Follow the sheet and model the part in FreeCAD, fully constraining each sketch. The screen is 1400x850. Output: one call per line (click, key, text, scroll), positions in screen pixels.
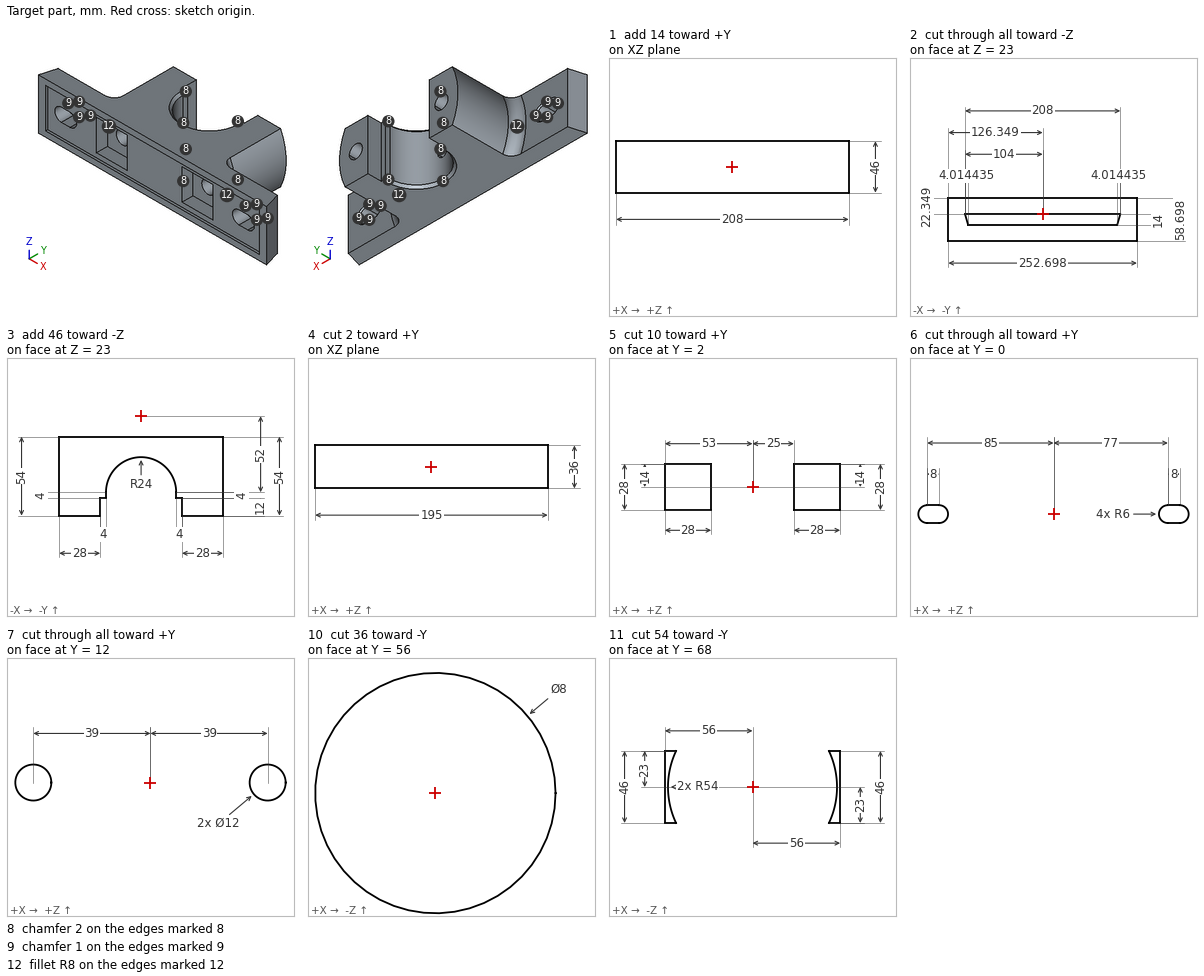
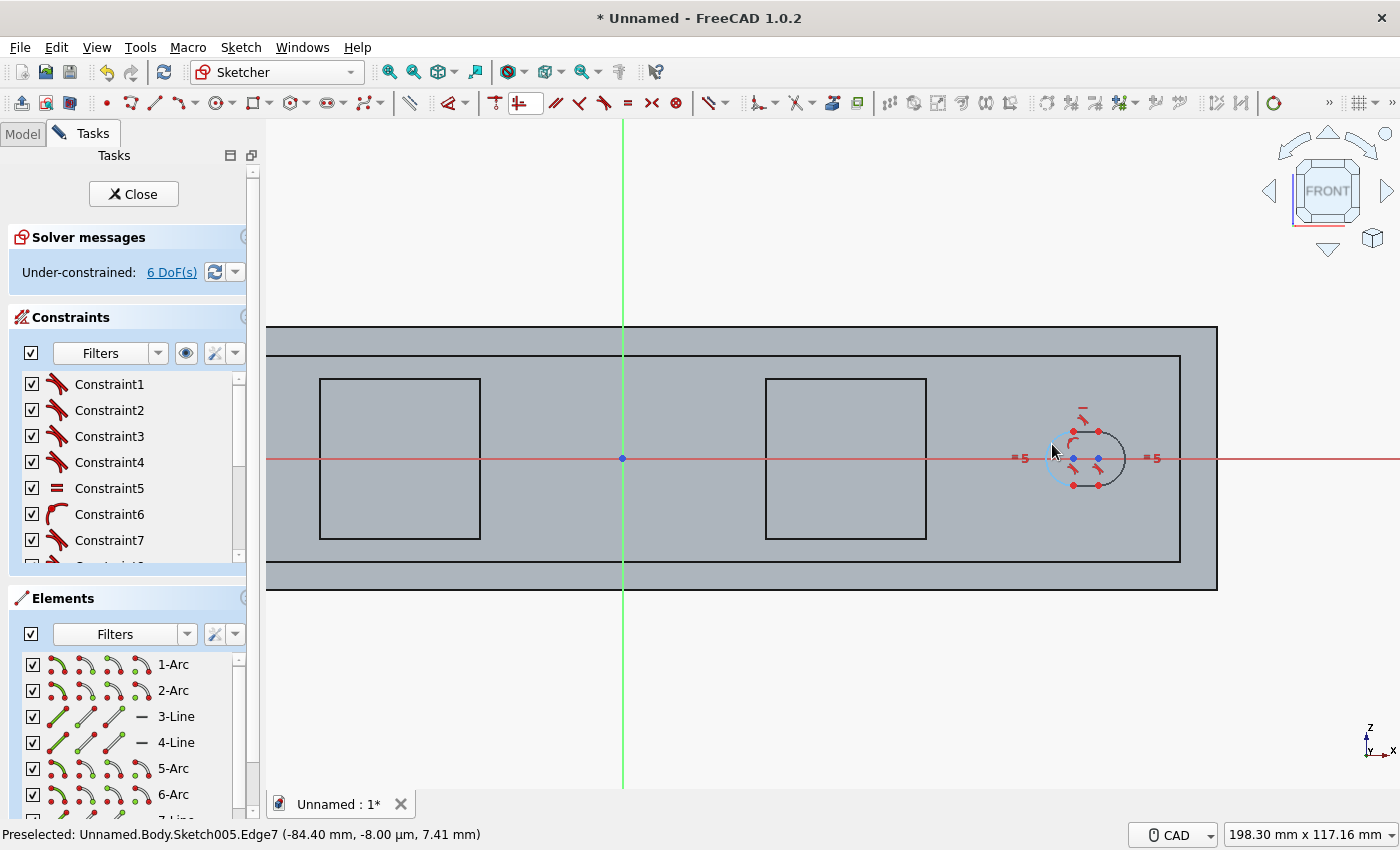
click(1051, 443)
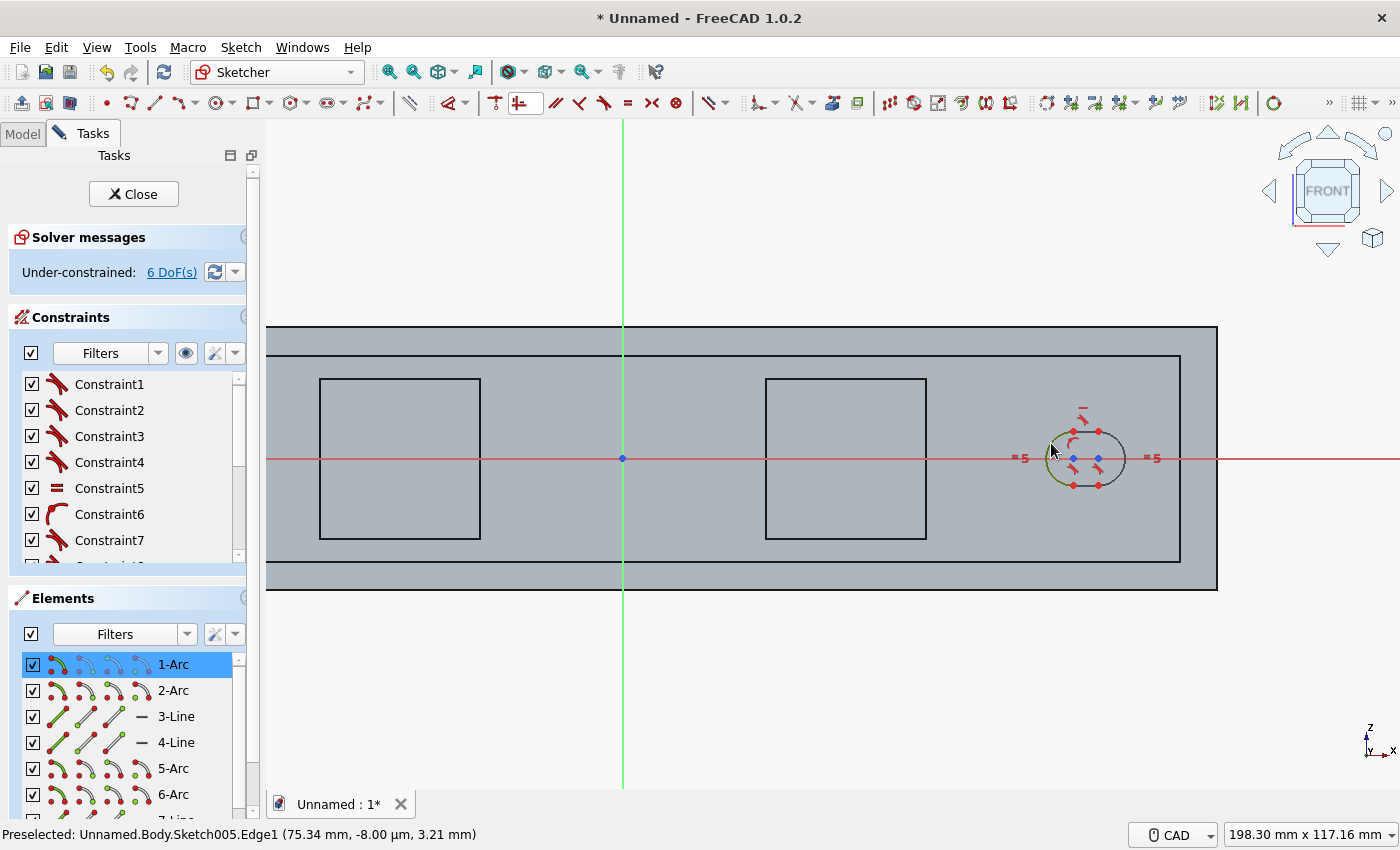
scroll(1053, 444, down, 2)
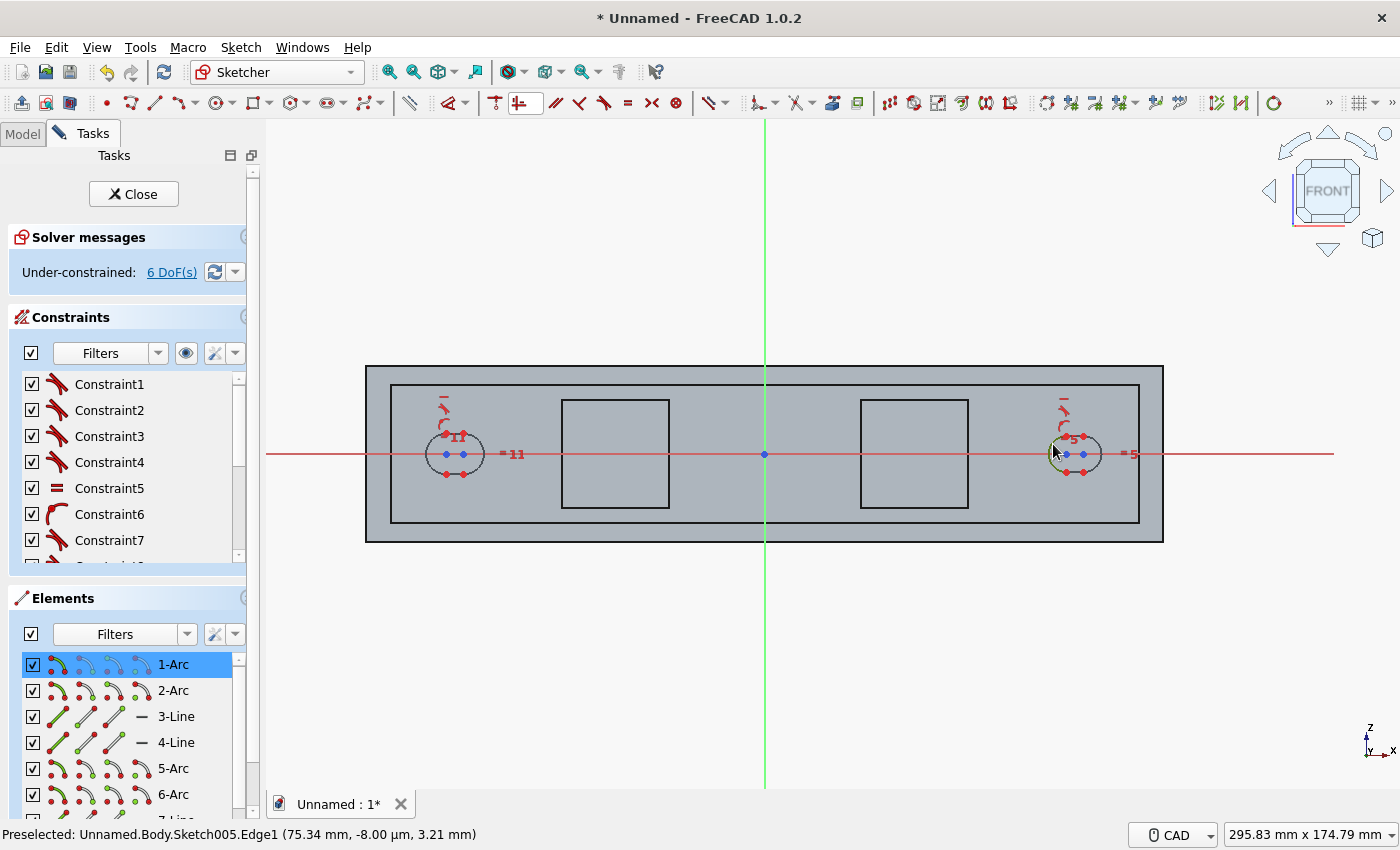
click(430, 442)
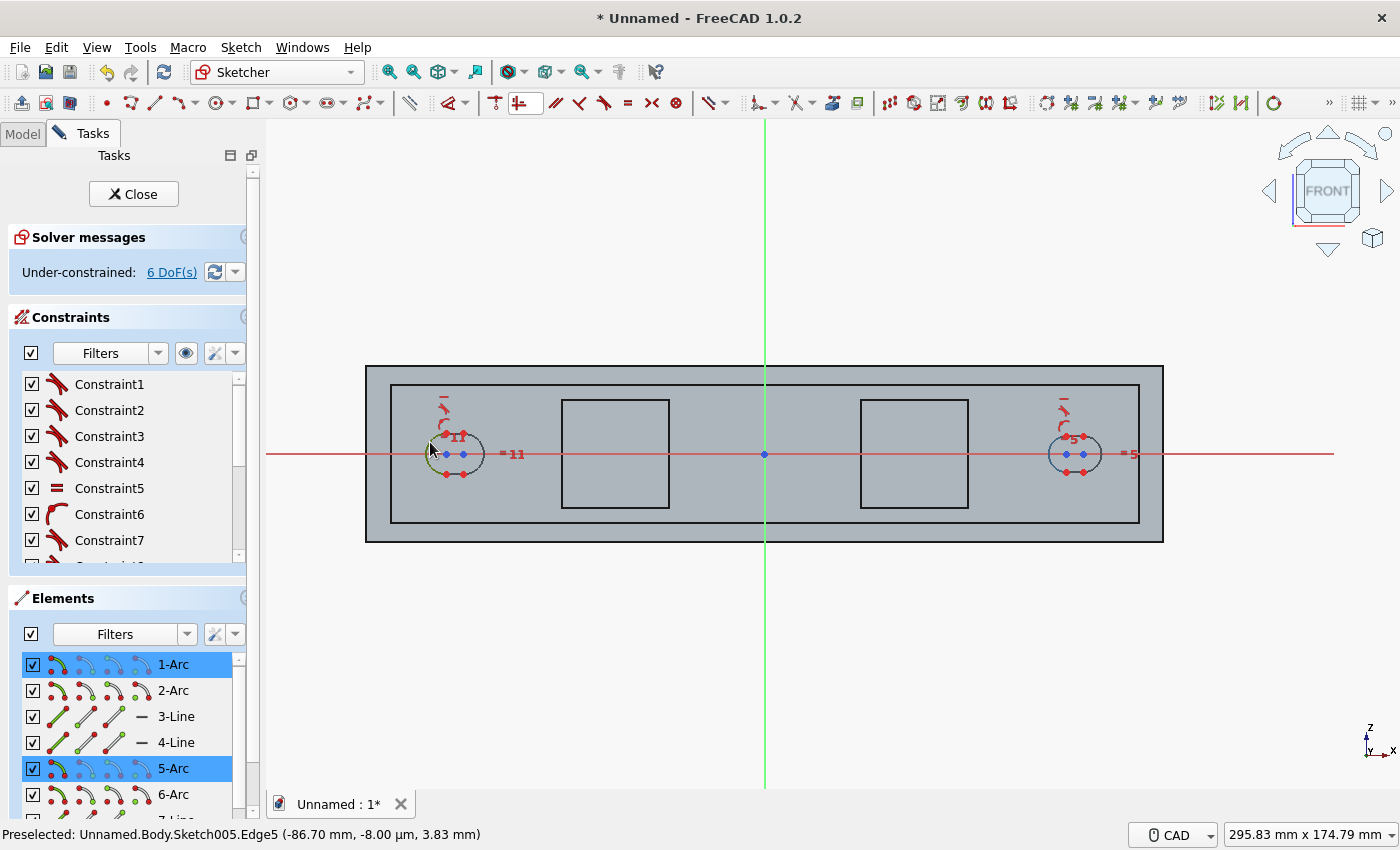
key(e)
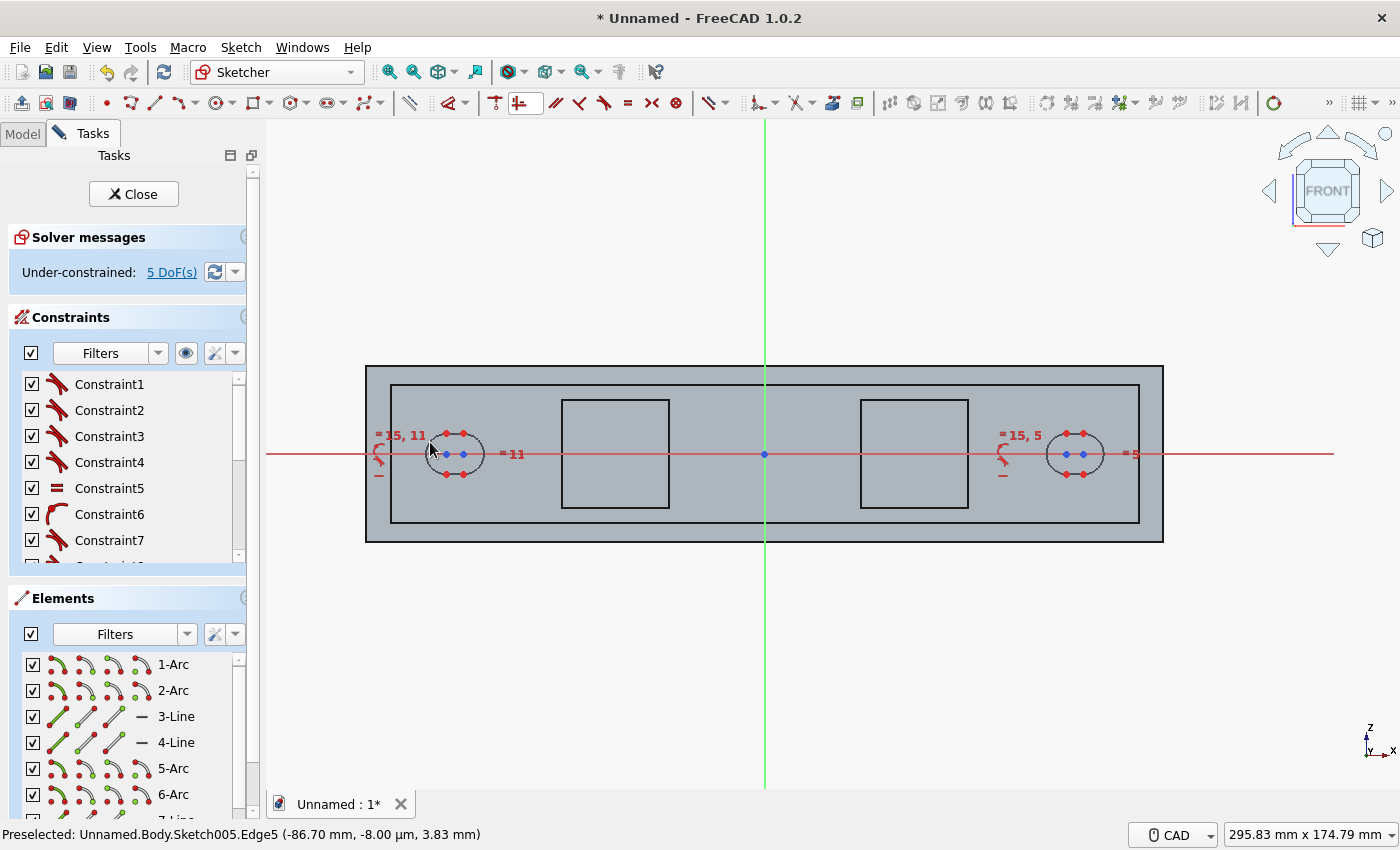
key(d)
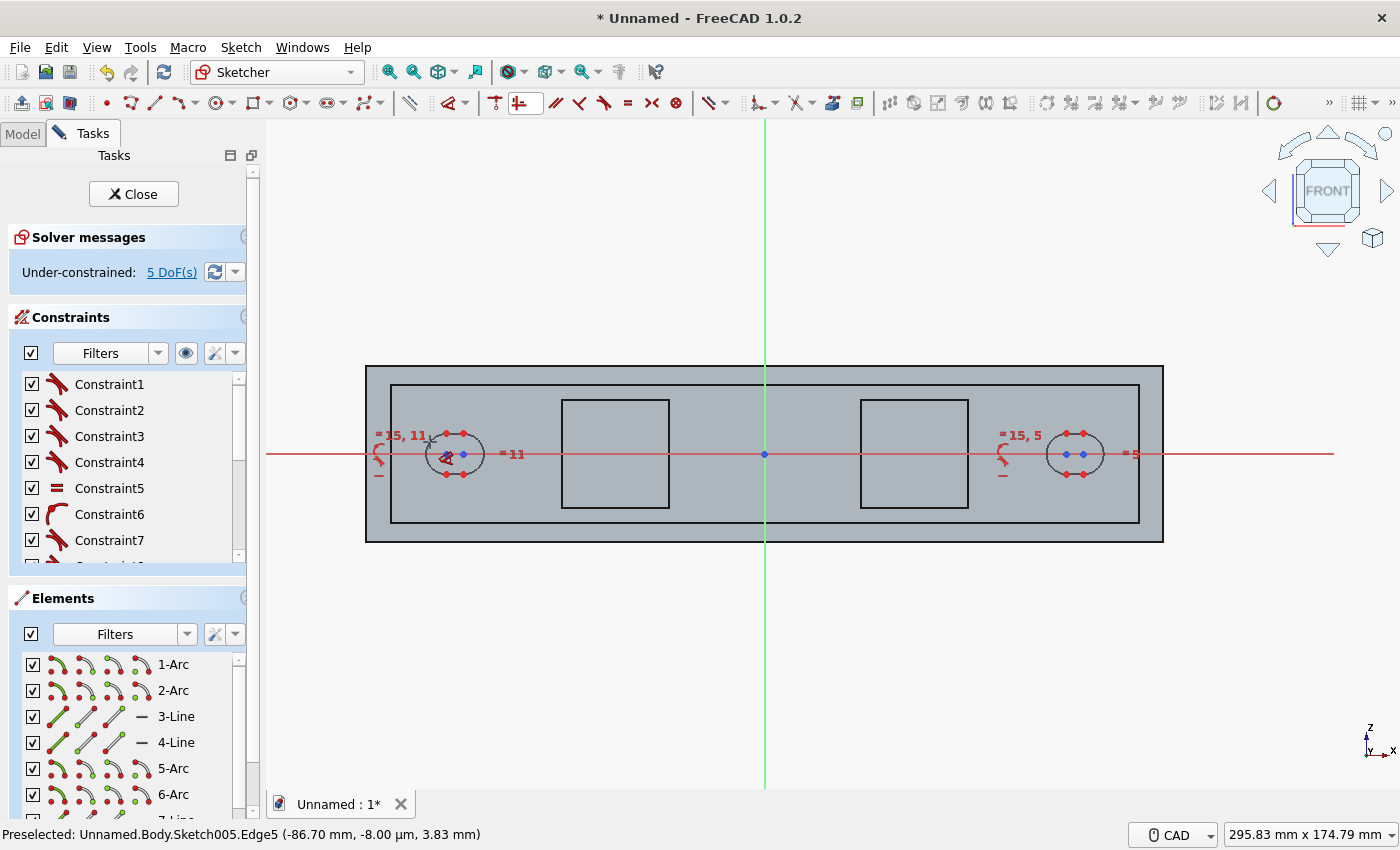
scroll(1050, 442, up, 3)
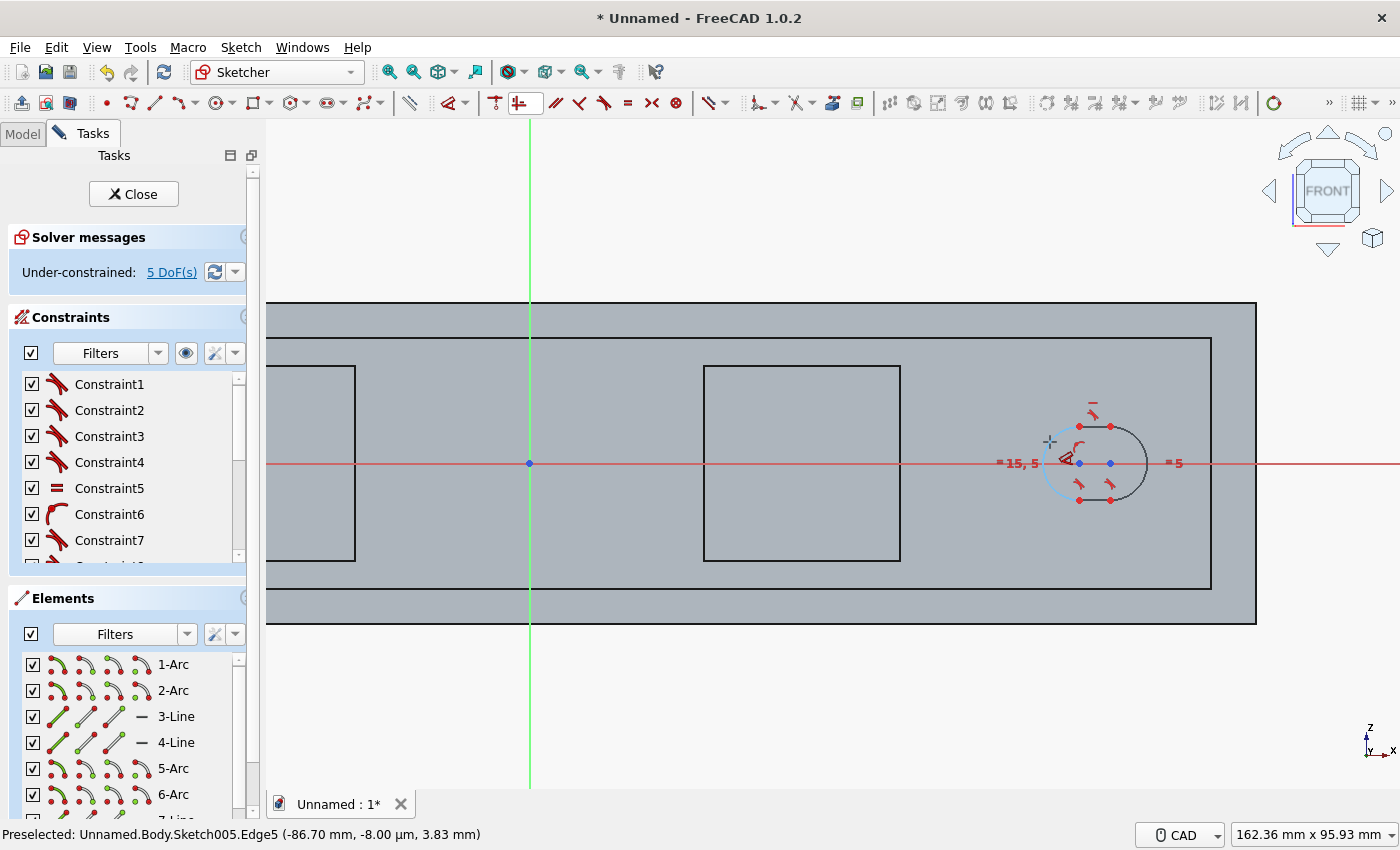
click(1050, 442)
click(1024, 423)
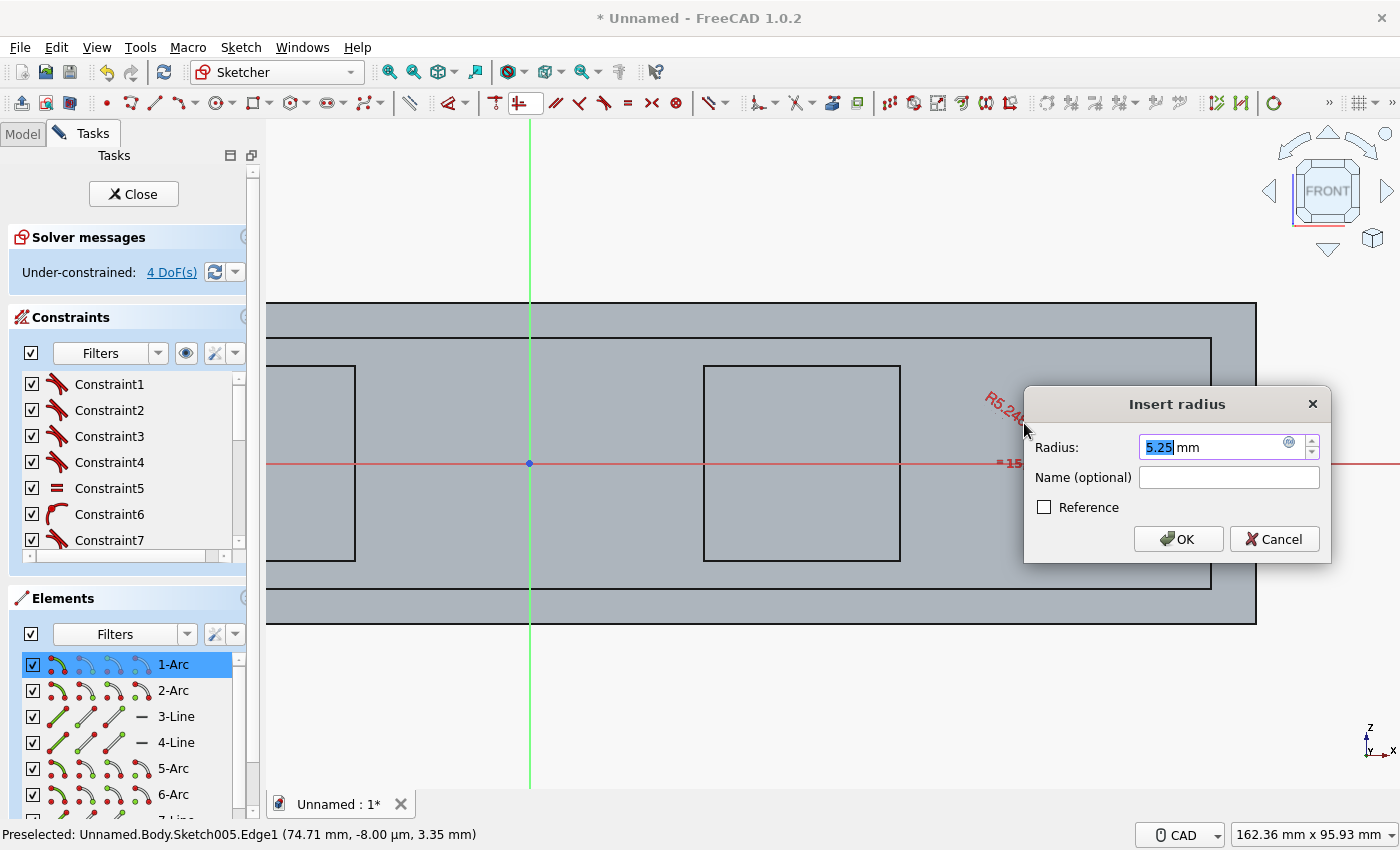
text(6)
key(Return)